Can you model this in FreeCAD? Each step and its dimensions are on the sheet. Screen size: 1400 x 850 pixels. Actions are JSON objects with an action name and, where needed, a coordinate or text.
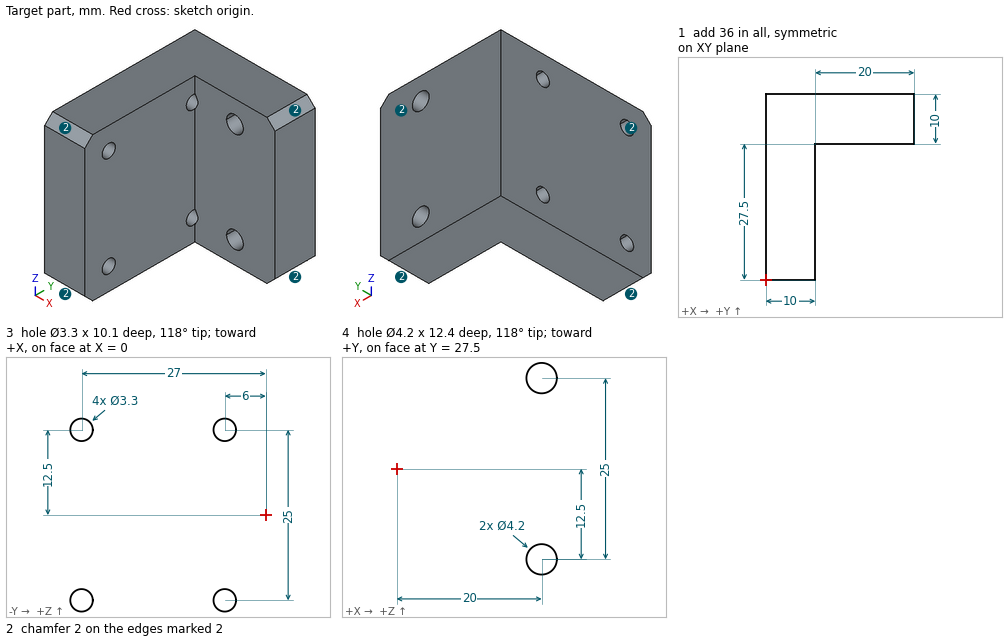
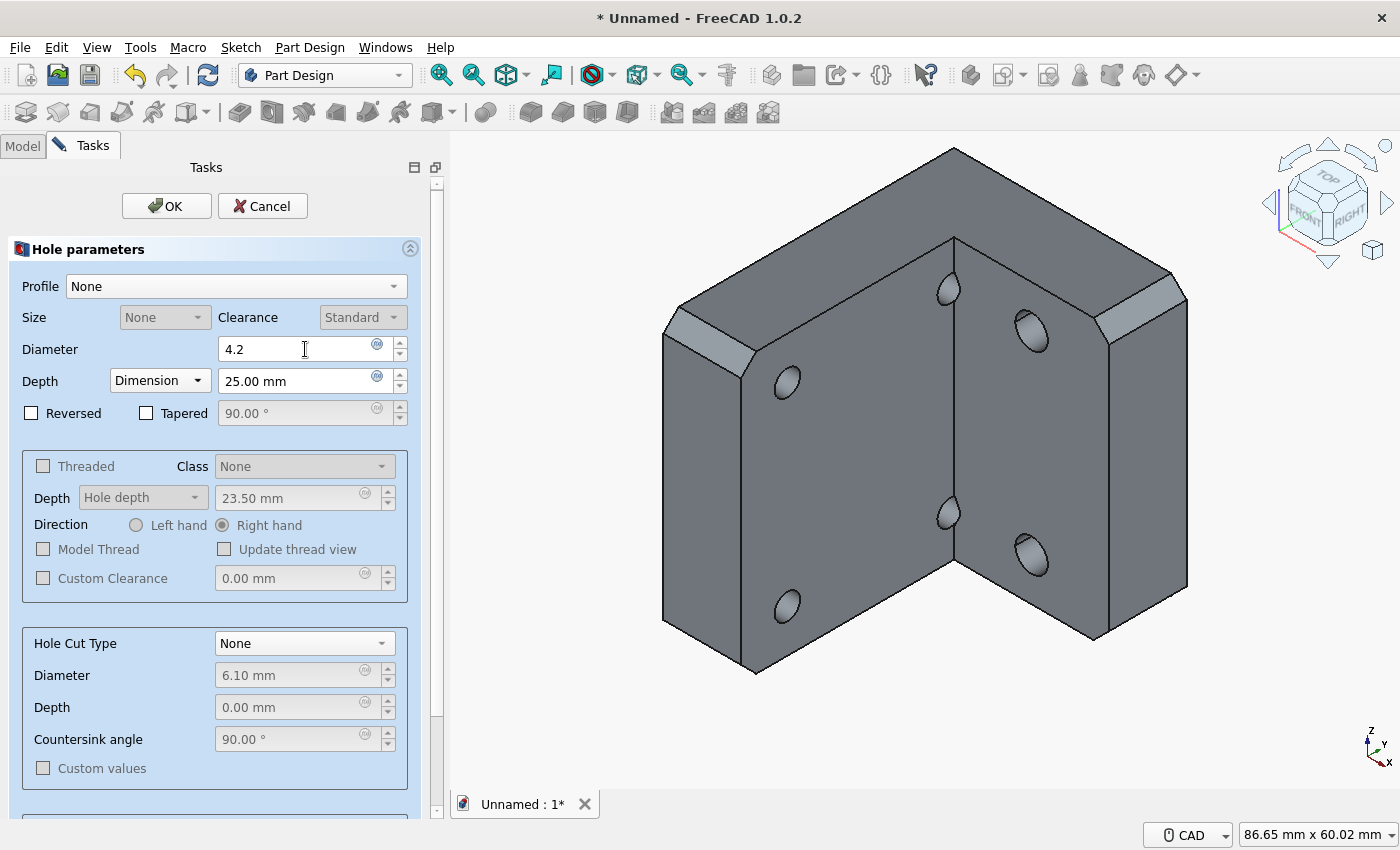
{"action": "triple_click", "coordinate": [305, 381]}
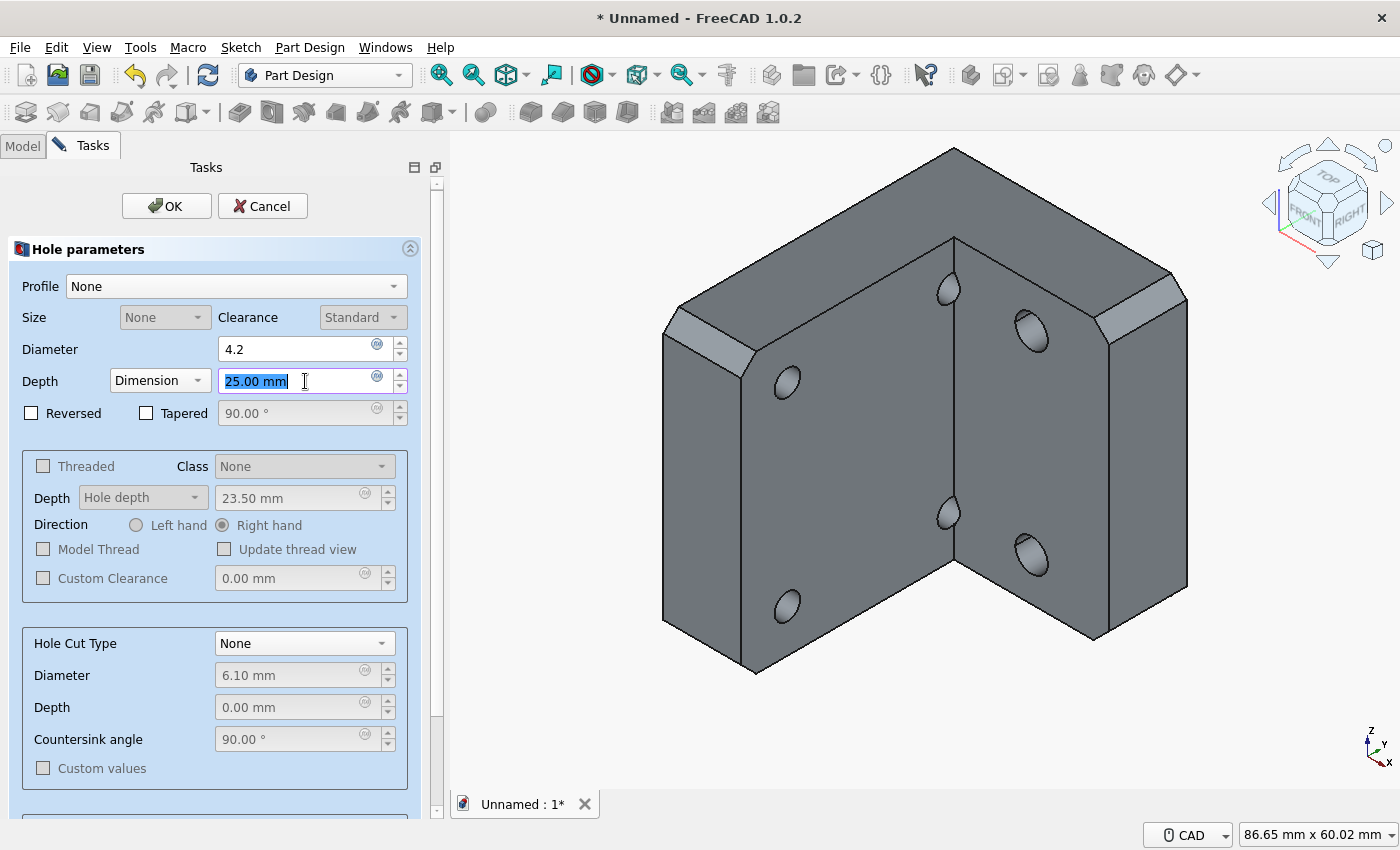
{"action": "type", "text": "12.4"}
{"action": "key", "text": "Tab"}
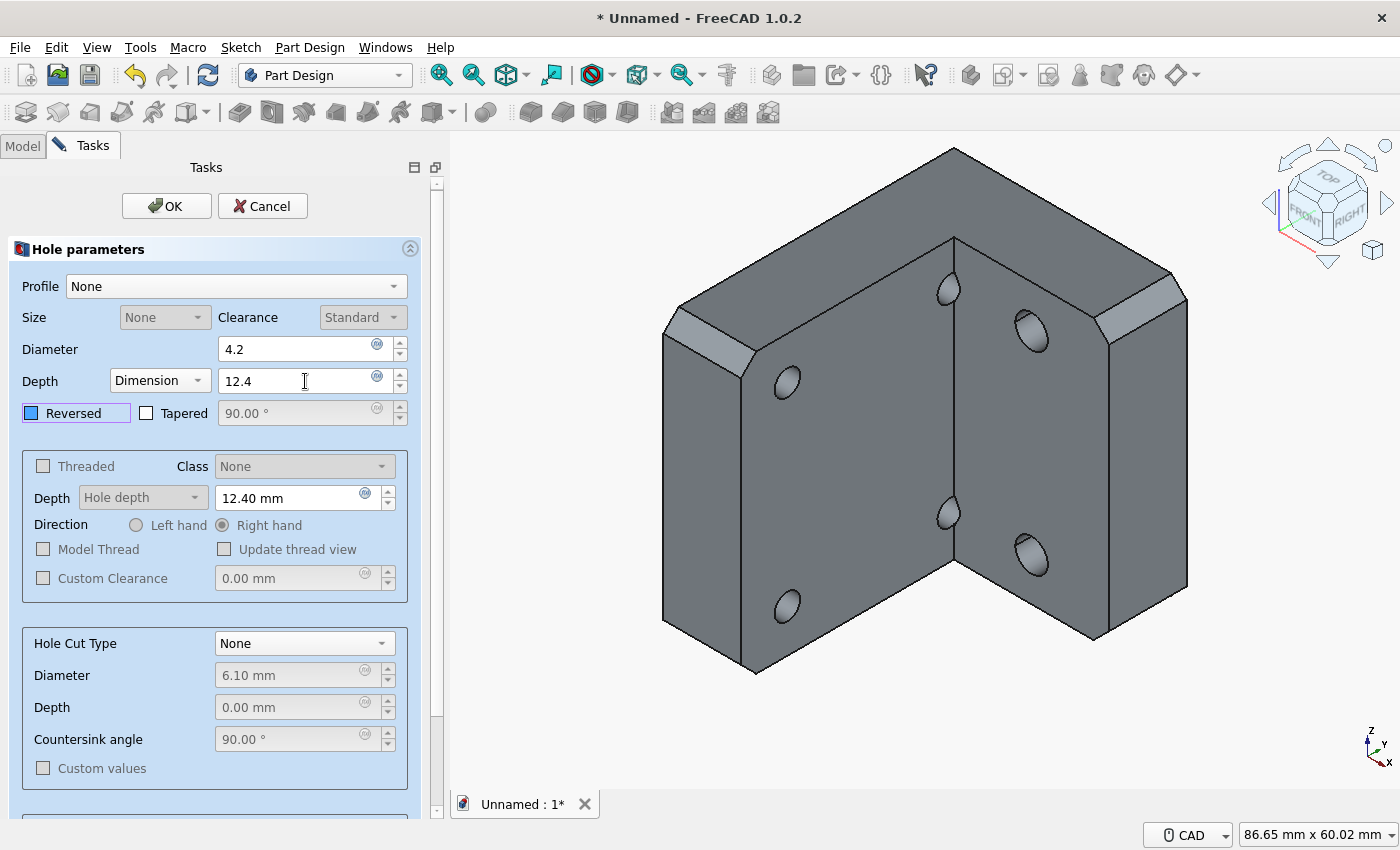
{"action": "left_click", "coordinate": [167, 206]}